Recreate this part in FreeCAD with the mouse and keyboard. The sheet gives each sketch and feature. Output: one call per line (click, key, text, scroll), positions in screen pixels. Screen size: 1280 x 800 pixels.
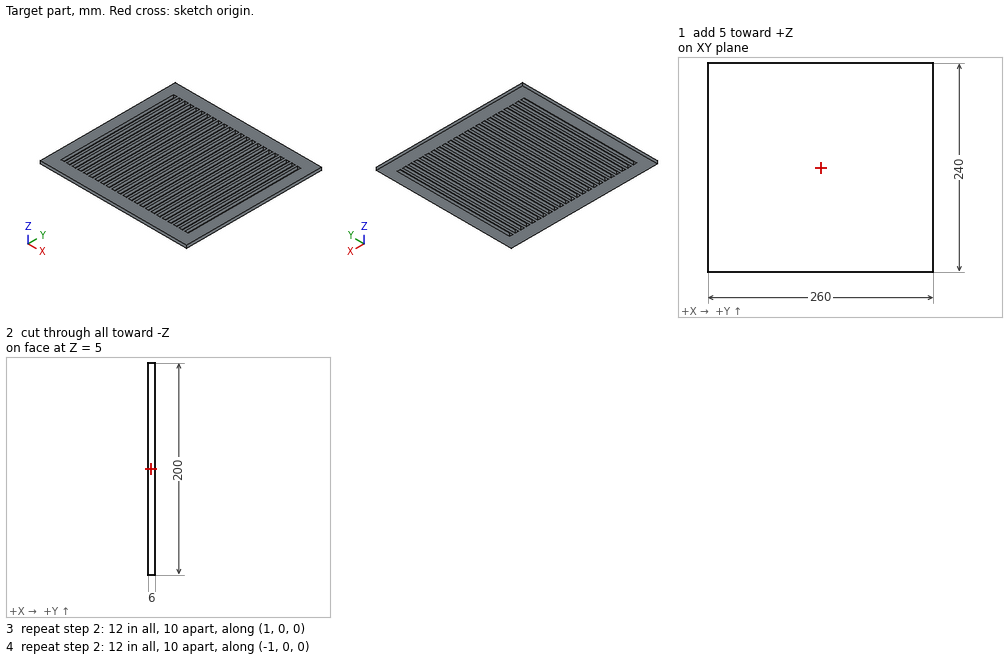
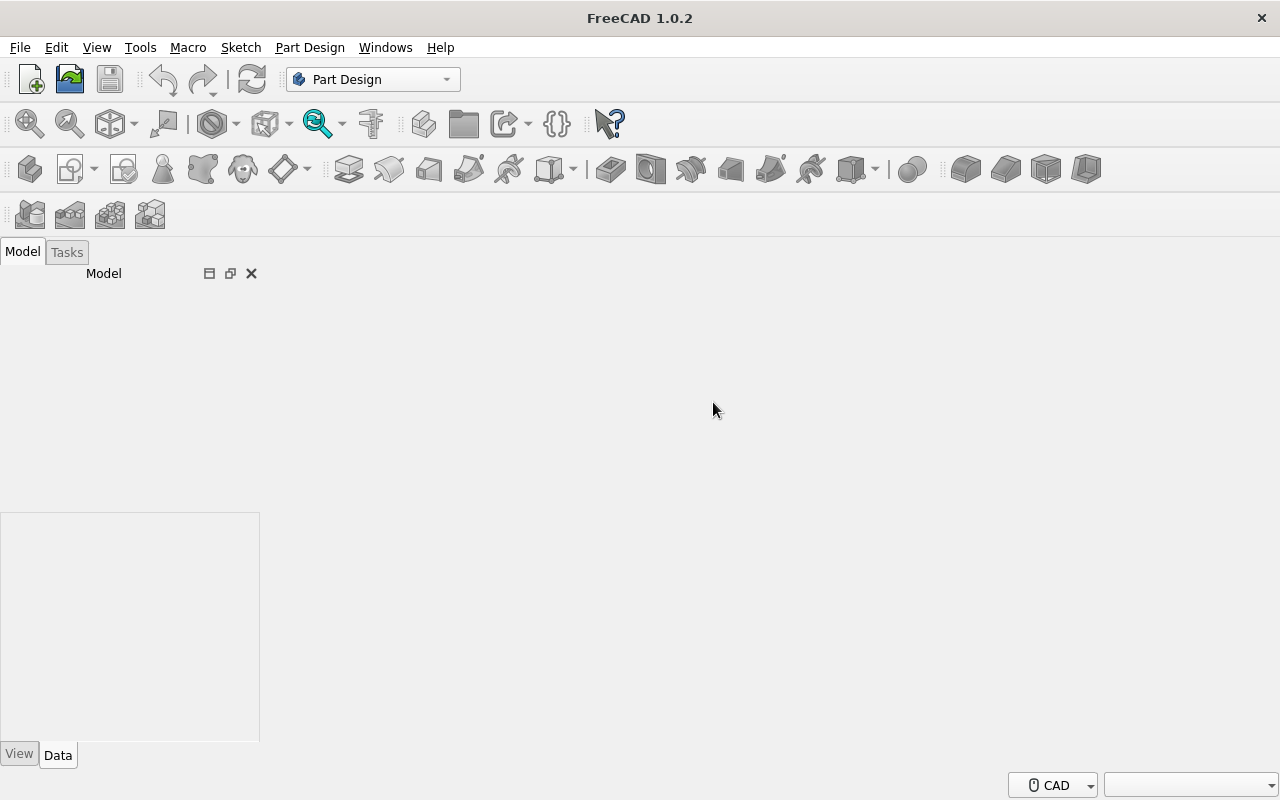
click(30, 80)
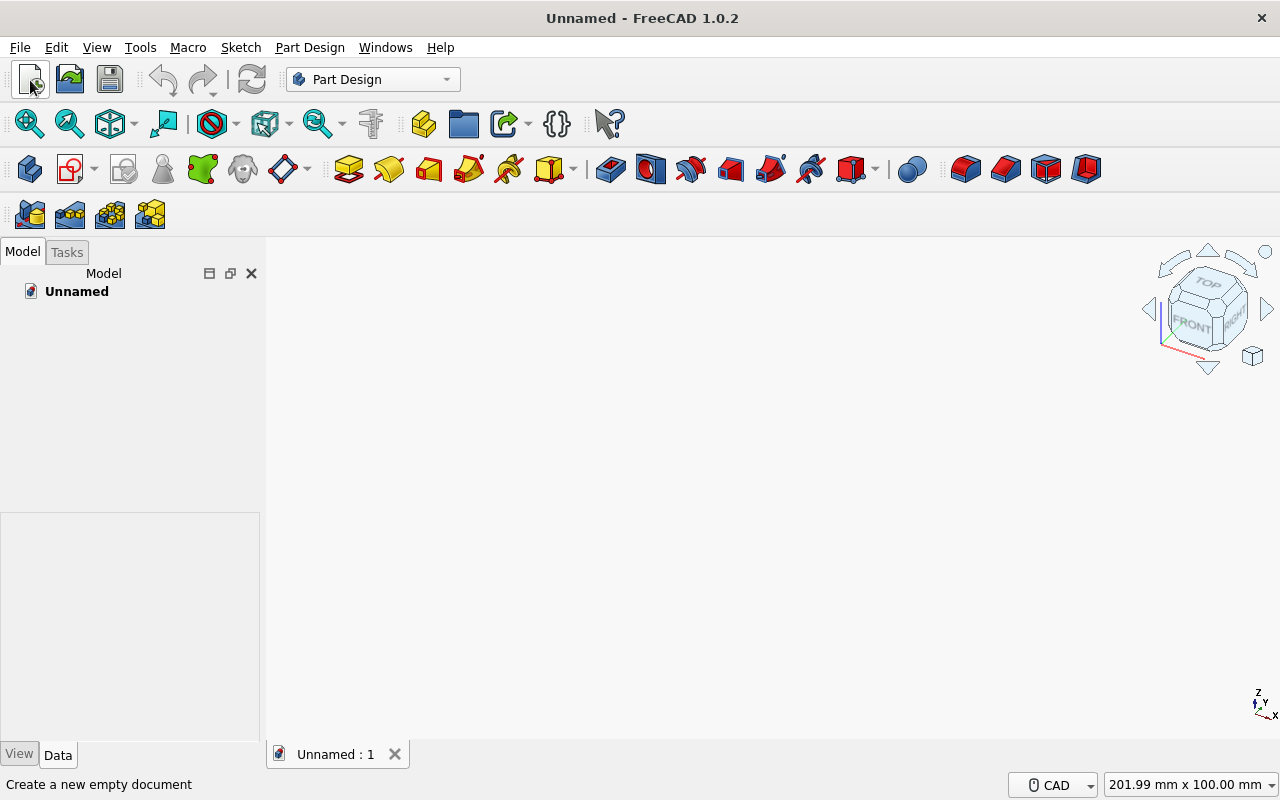
click(70, 170)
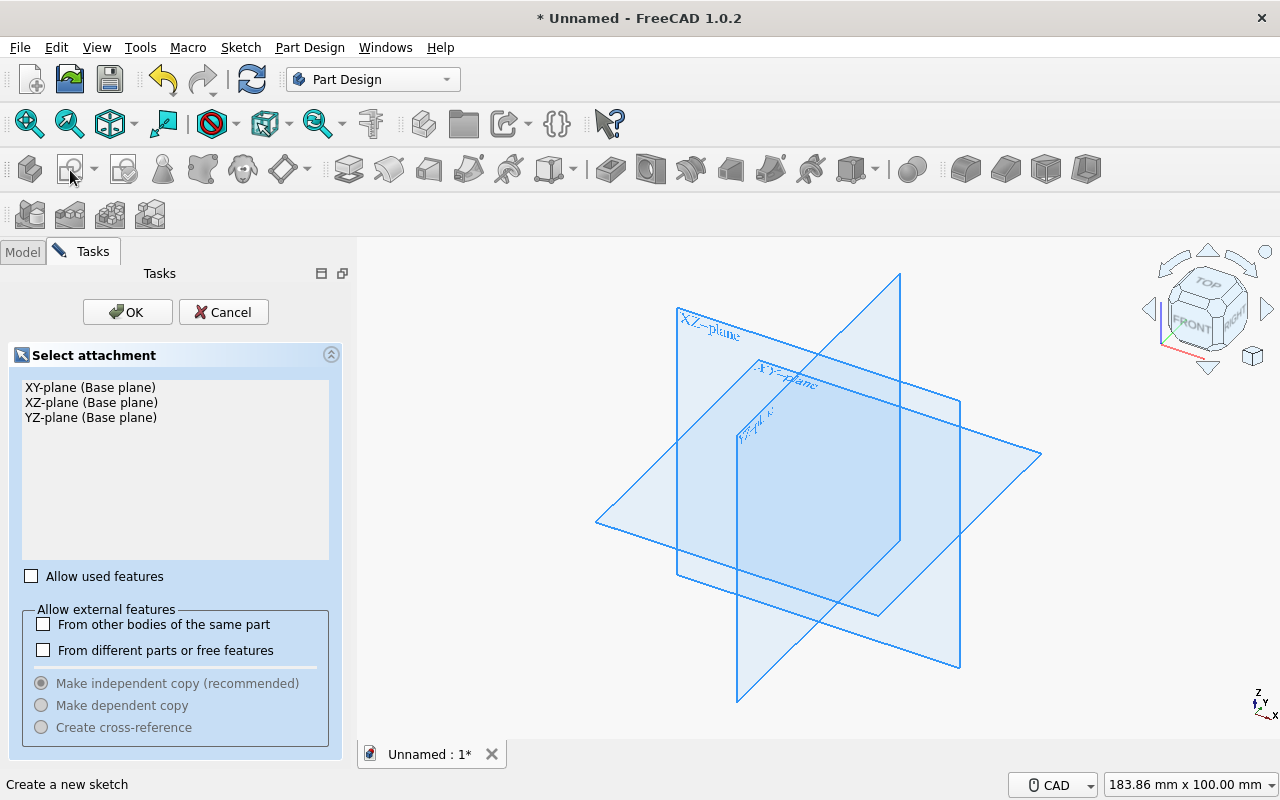
click(82, 388)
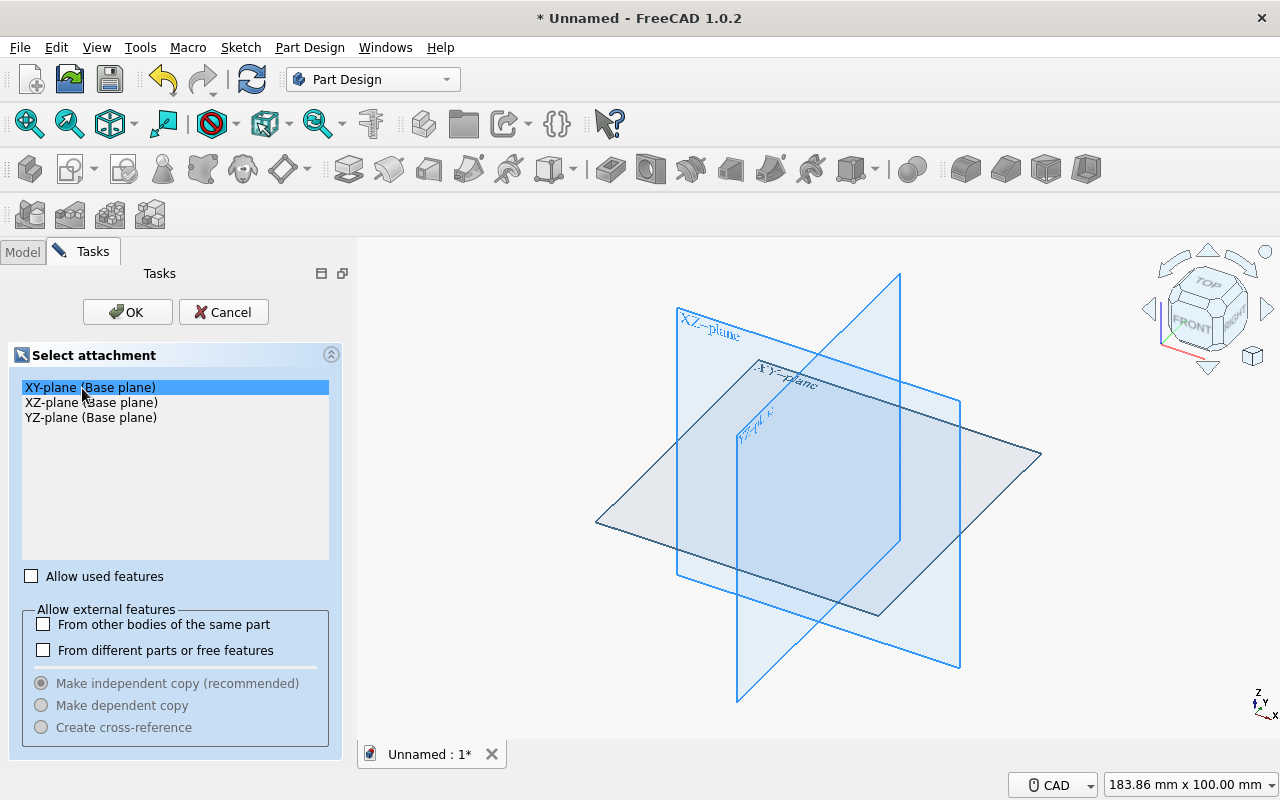
click(128, 312)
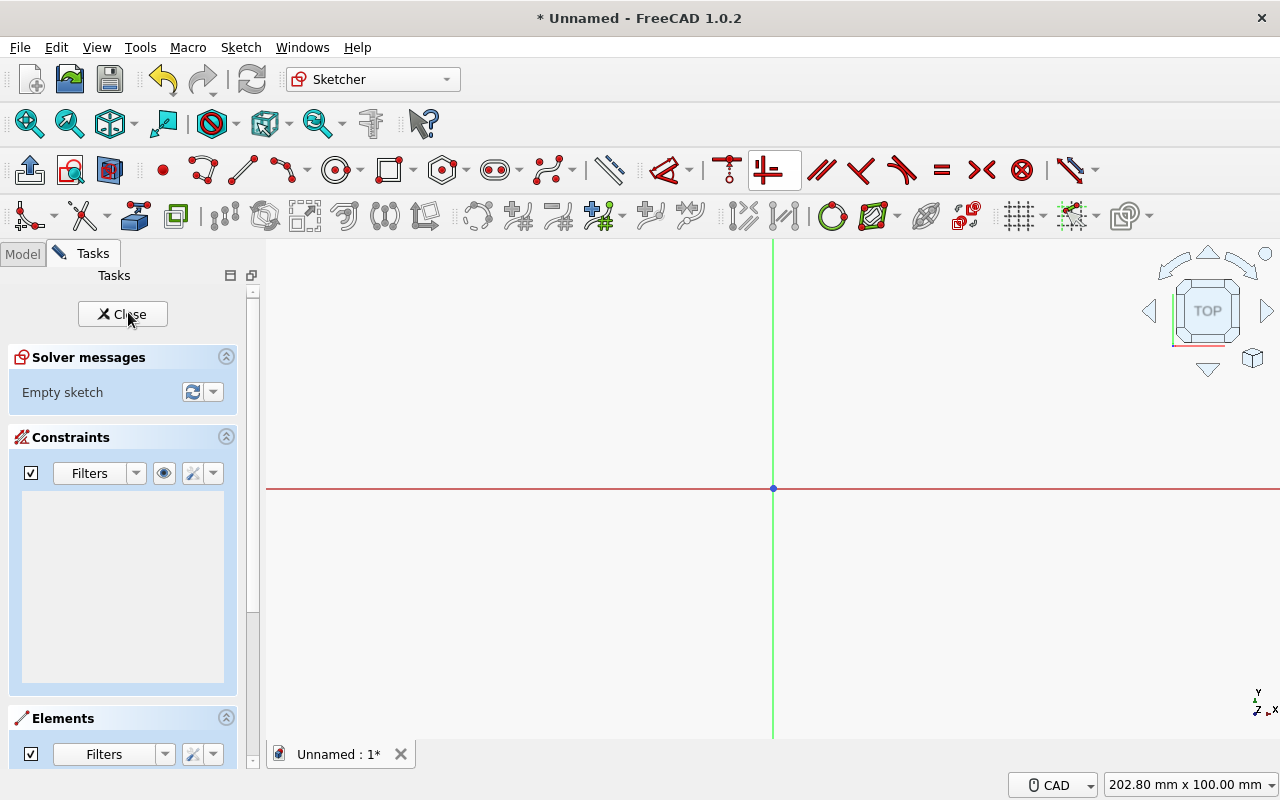
scroll(682, 489, down, 7)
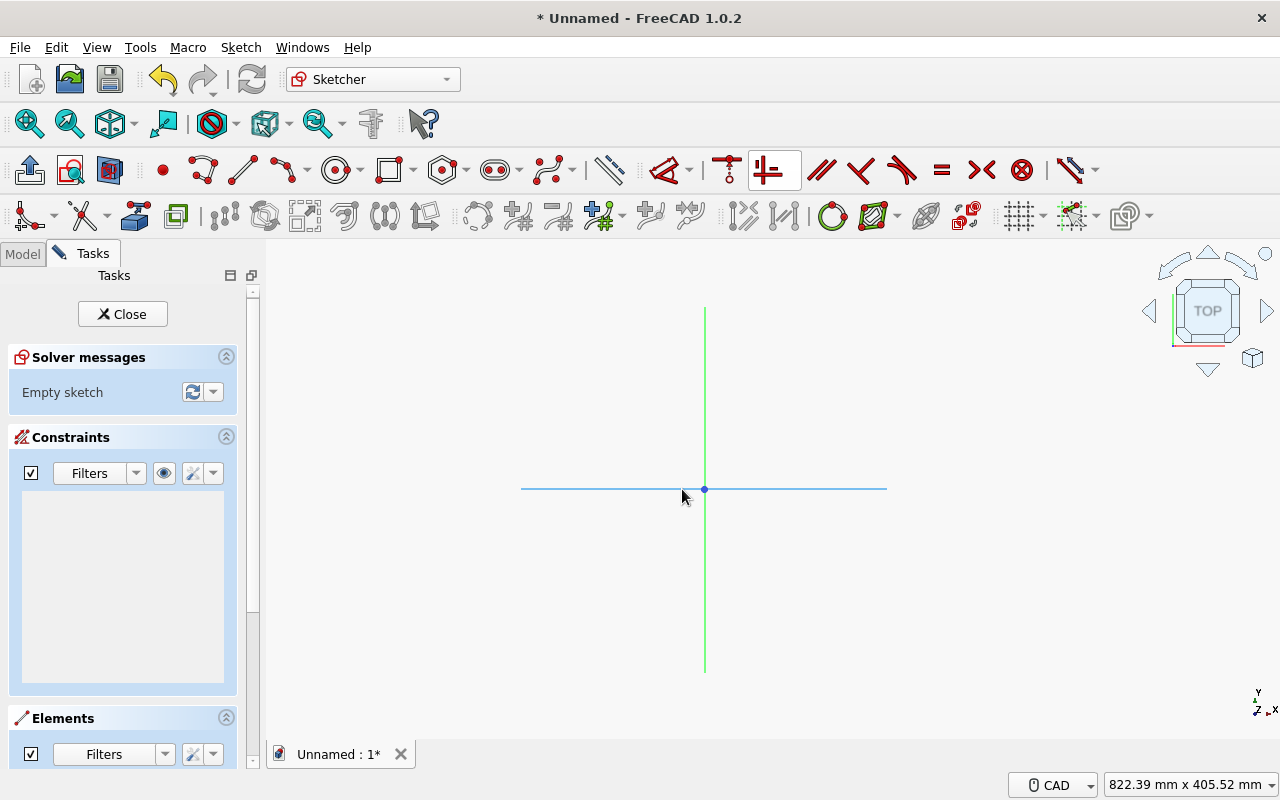
click(416, 170)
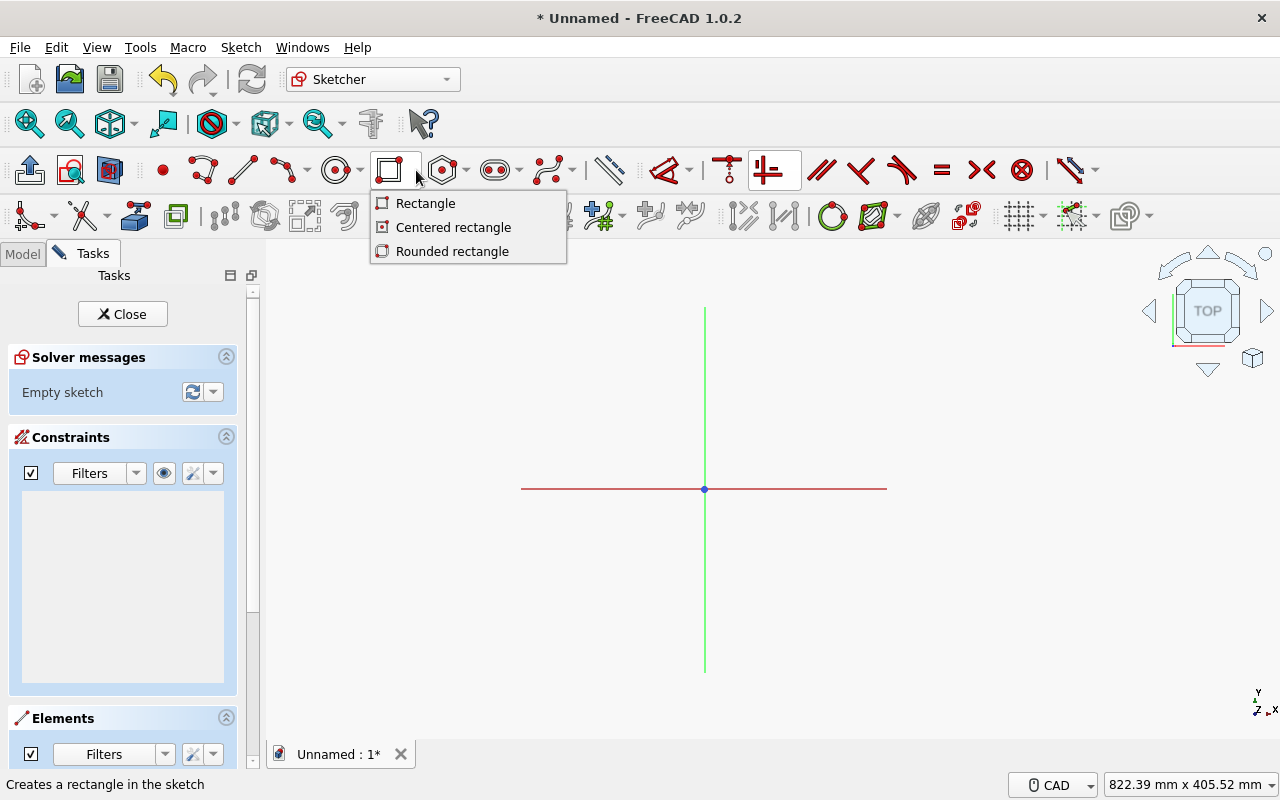
click(468, 227)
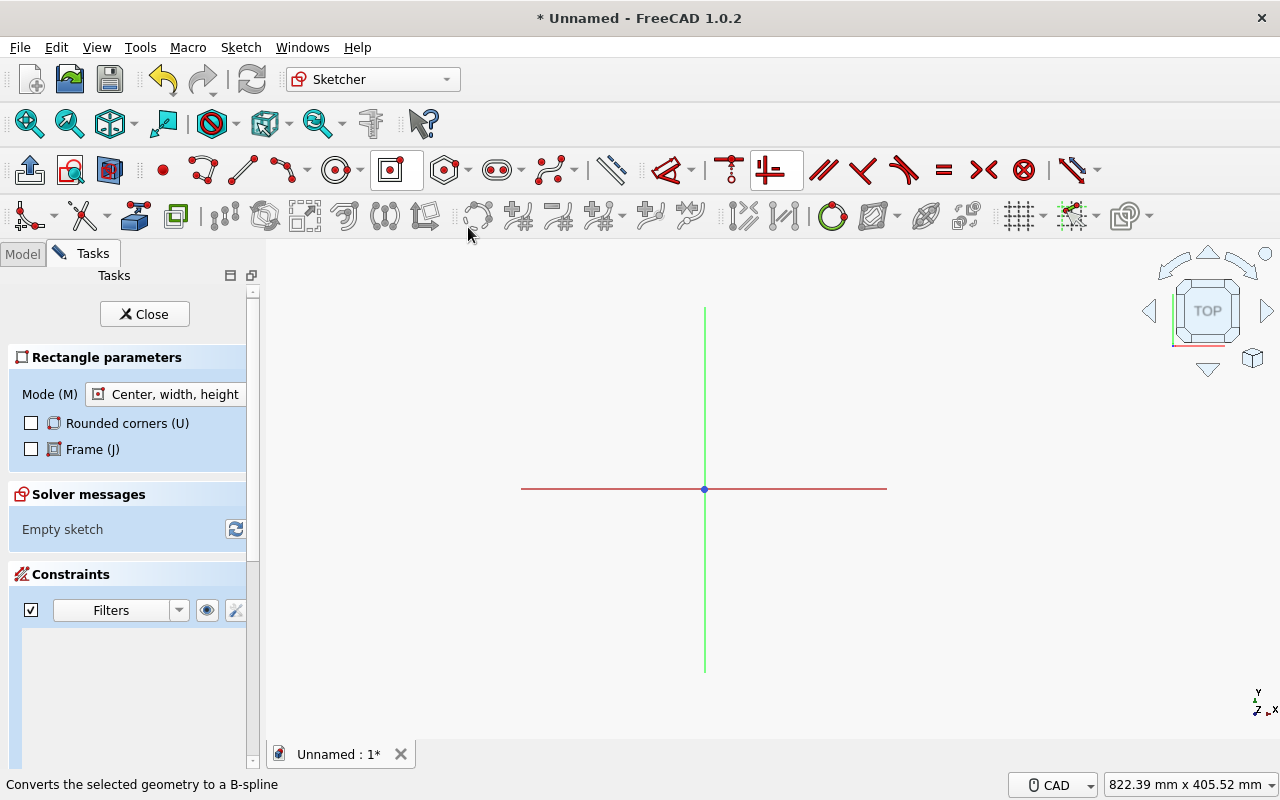
click(705, 489)
click(865, 341)
key(Escape)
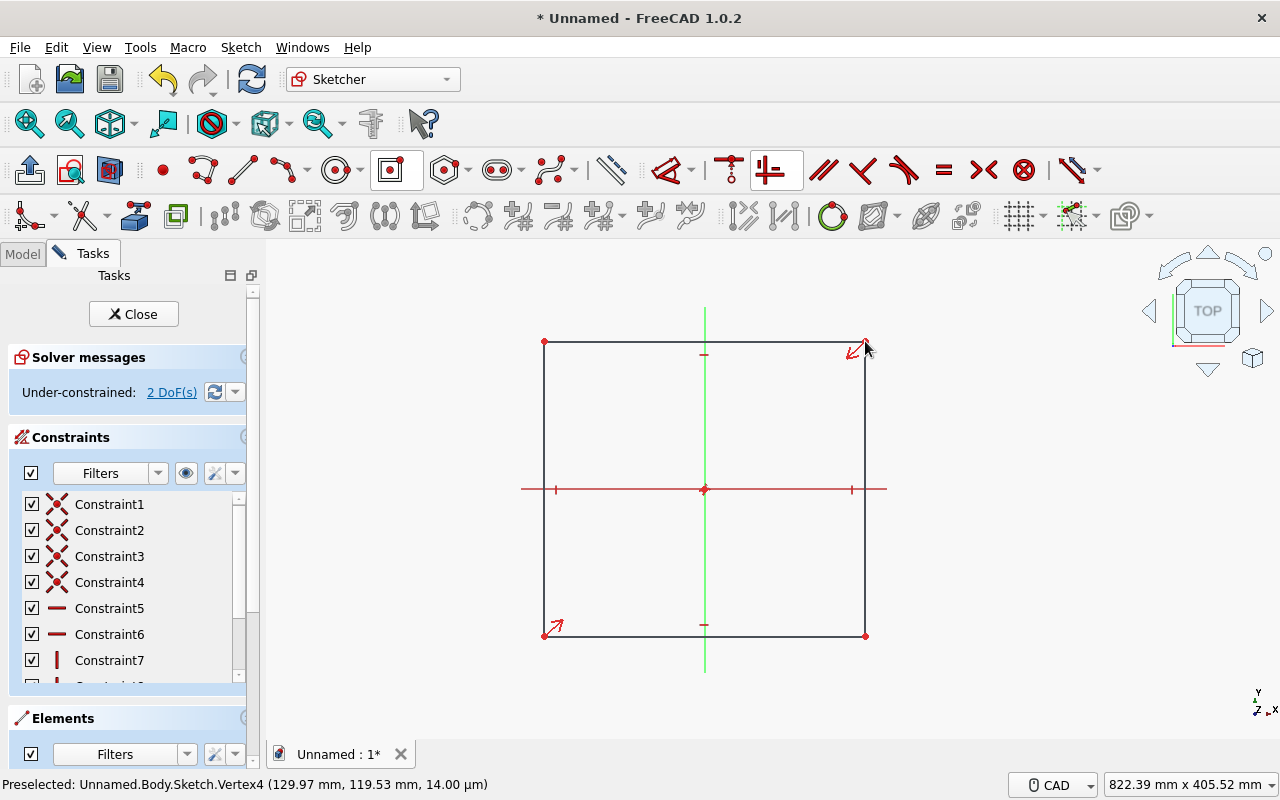
click(641, 637)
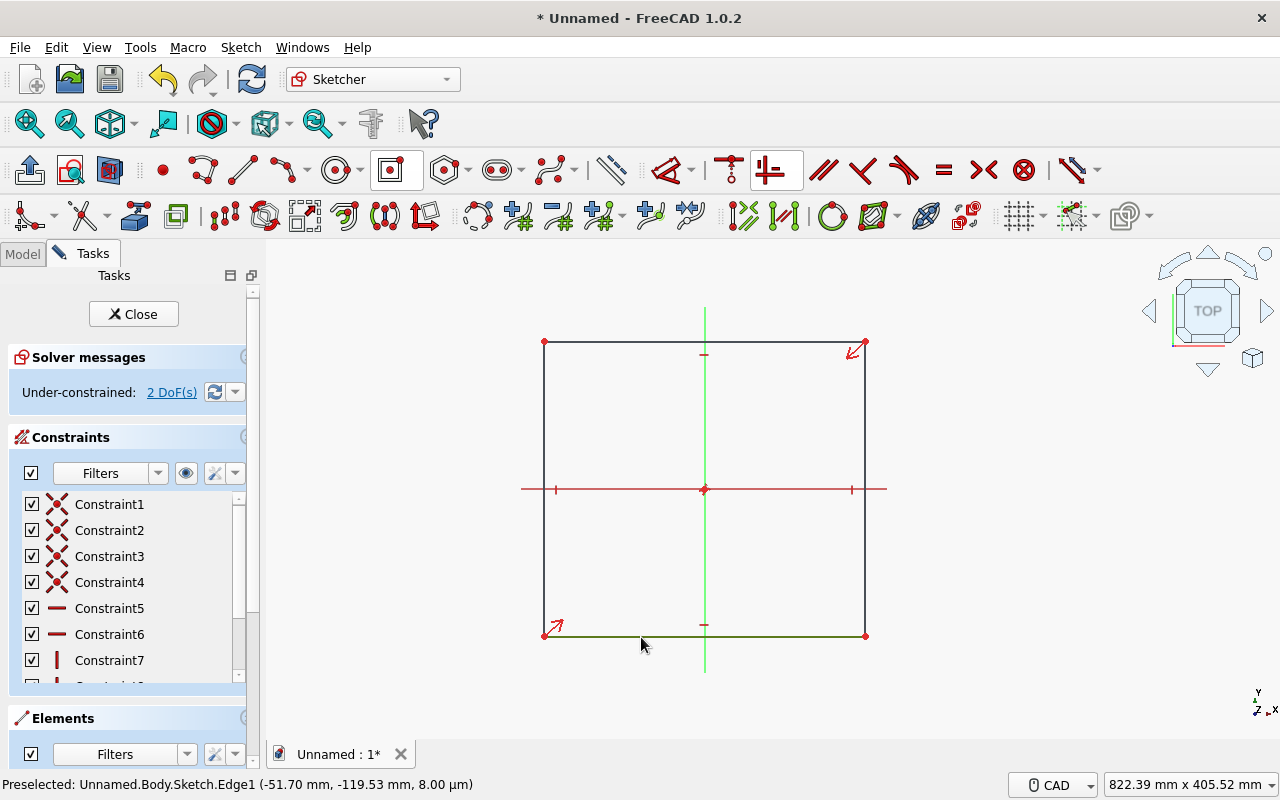
click(694, 170)